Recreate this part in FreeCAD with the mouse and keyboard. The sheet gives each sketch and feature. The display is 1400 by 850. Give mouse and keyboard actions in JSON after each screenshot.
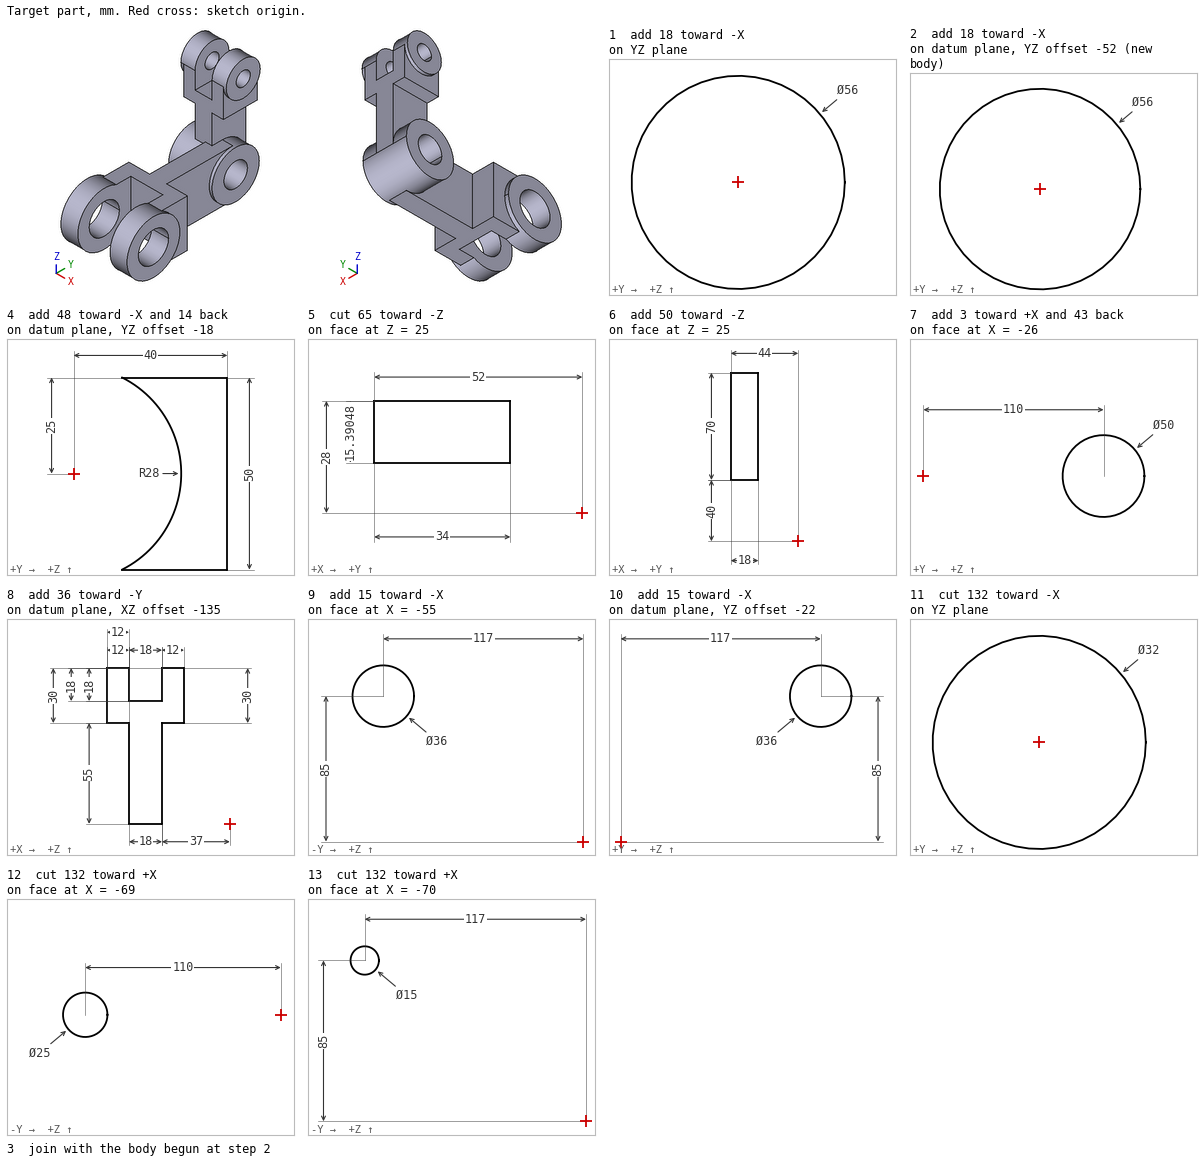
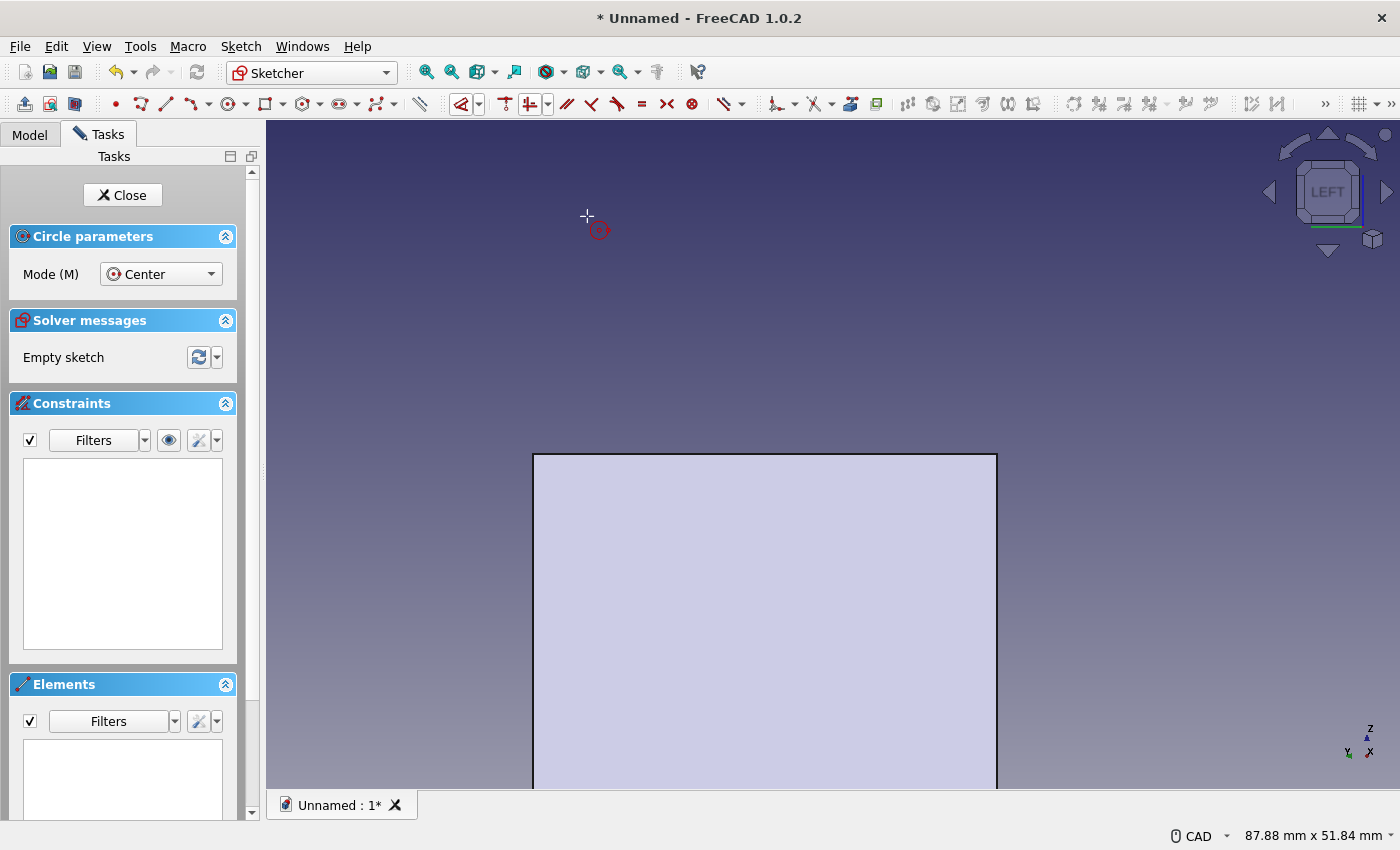
{"action": "left_click", "coordinate": [765, 454]}
{"action": "left_click", "coordinate": [929, 290]}
{"action": "key", "text": "Escape"}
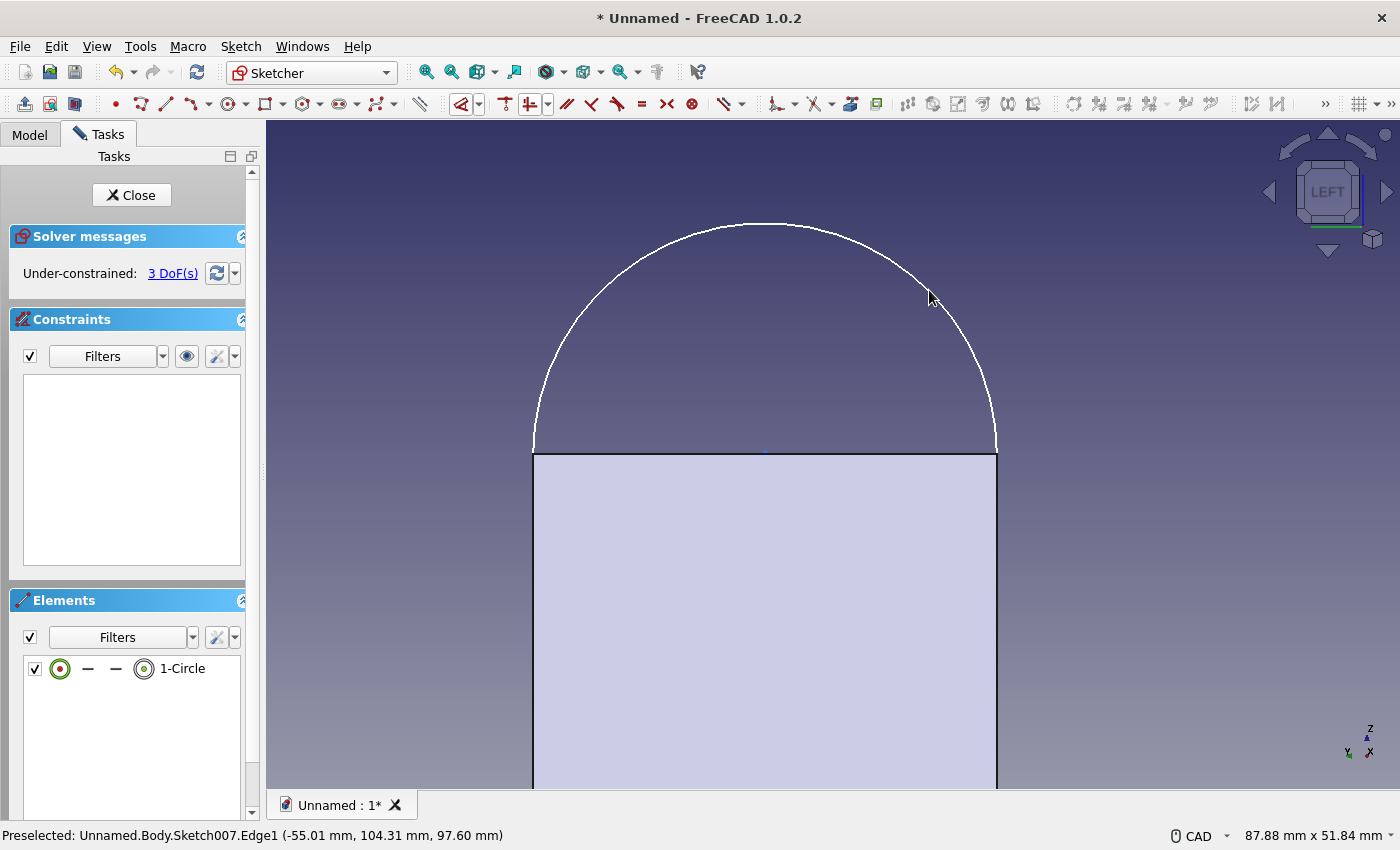
{"action": "left_click", "coordinate": [928, 290]}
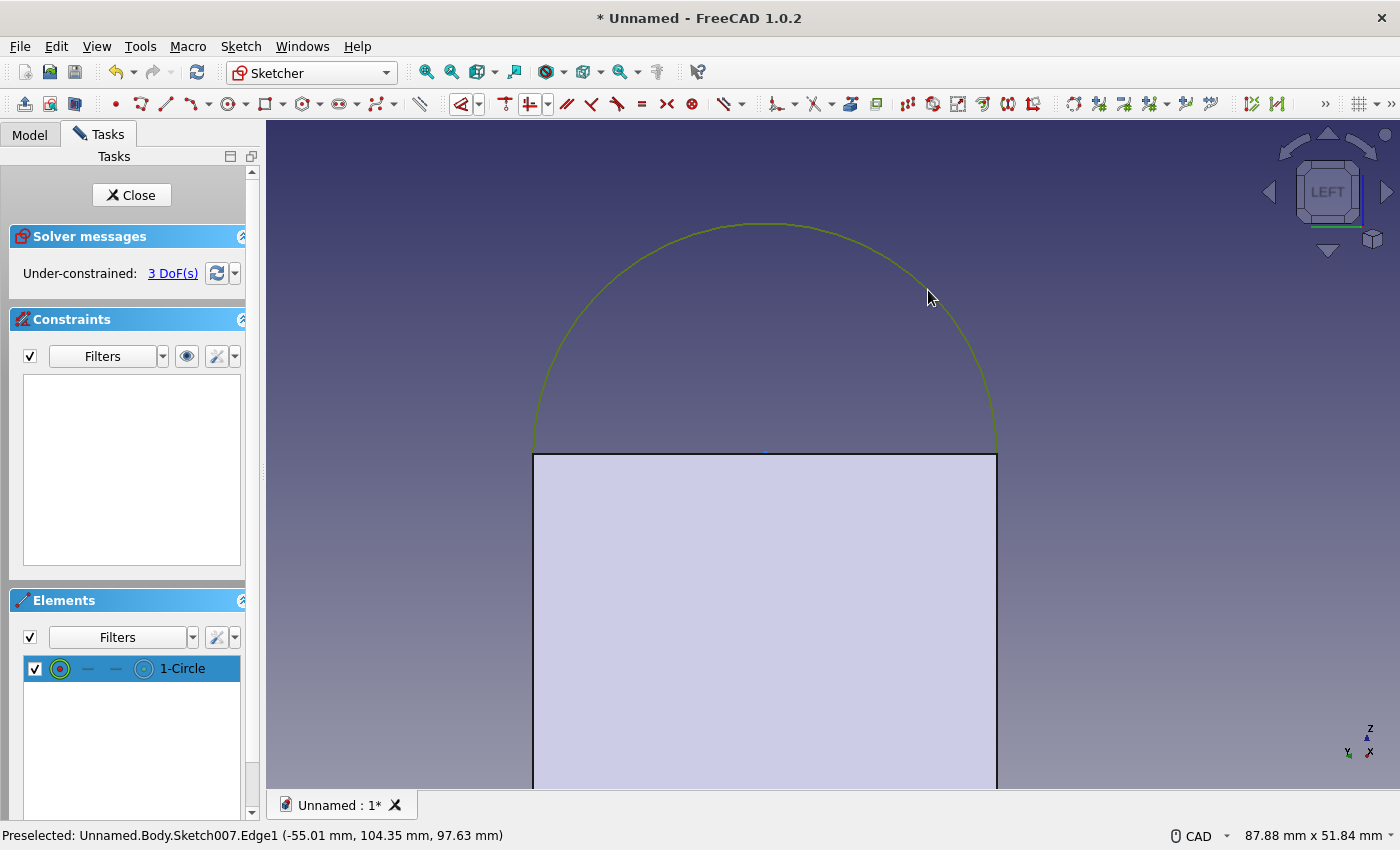
{"action": "key", "text": "k o"}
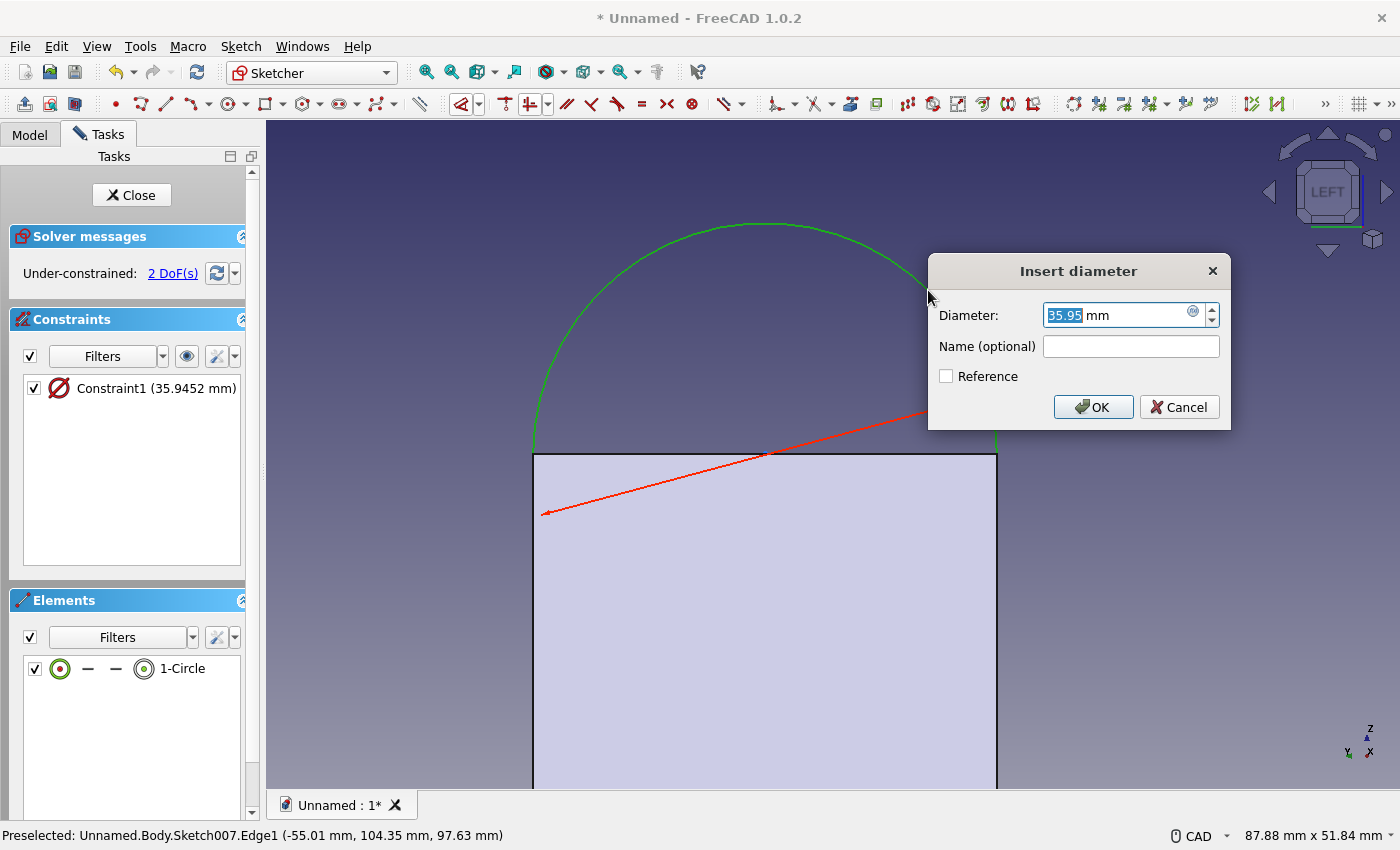
{"action": "type", "text": "36"}
{"action": "key", "text": "Return"}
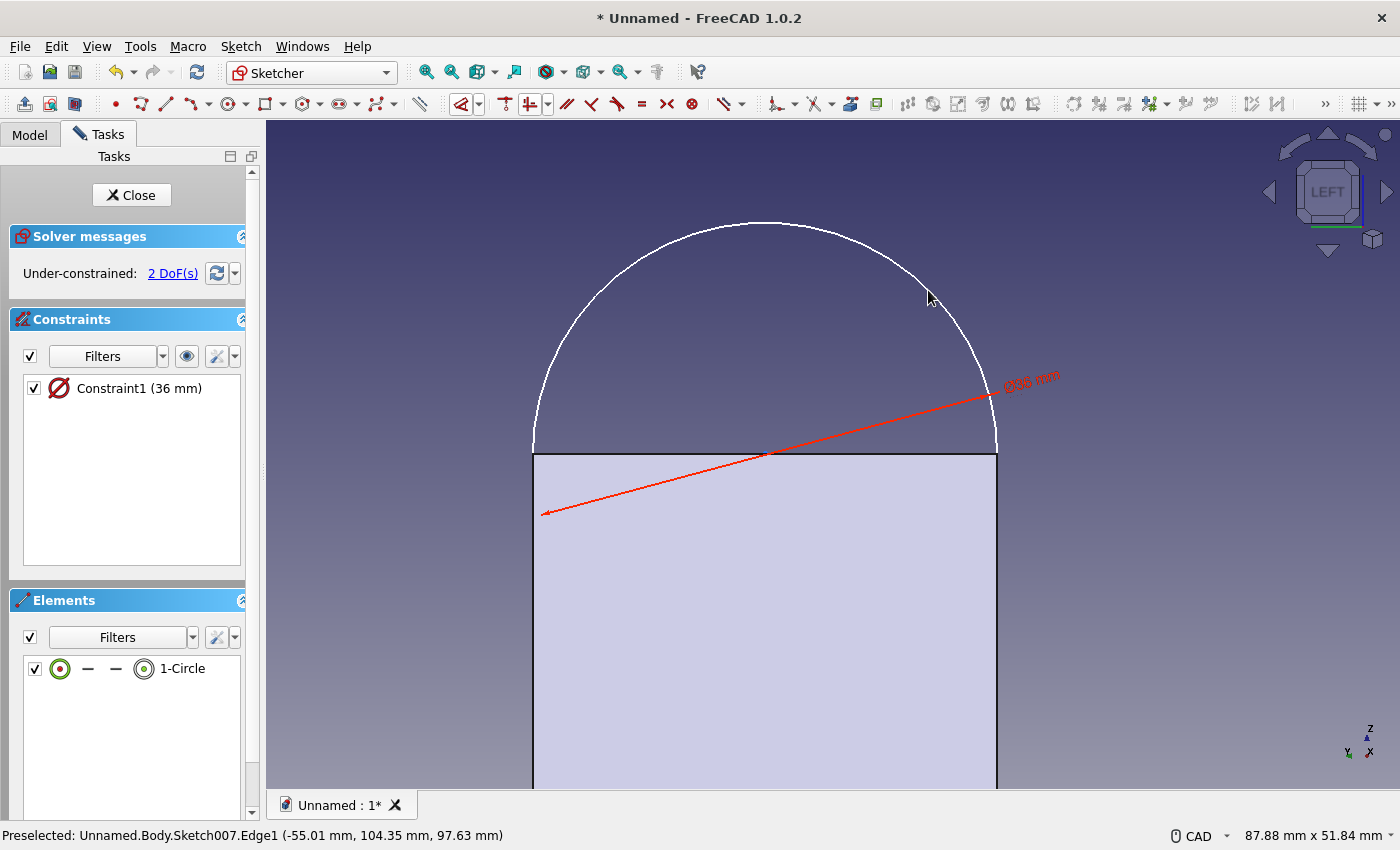
{"action": "left_click", "coordinate": [765, 455]}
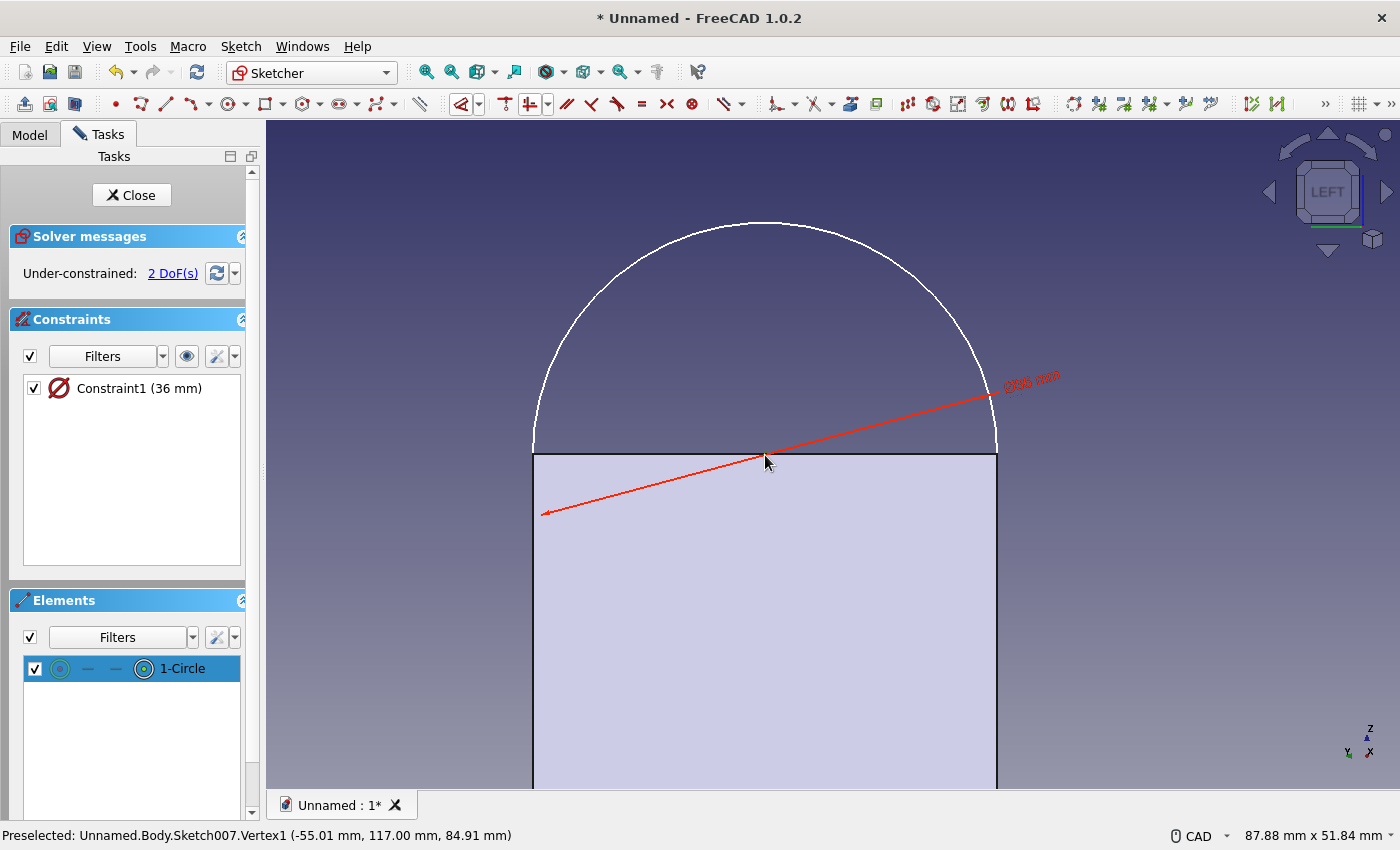
{"action": "key", "text": "i"}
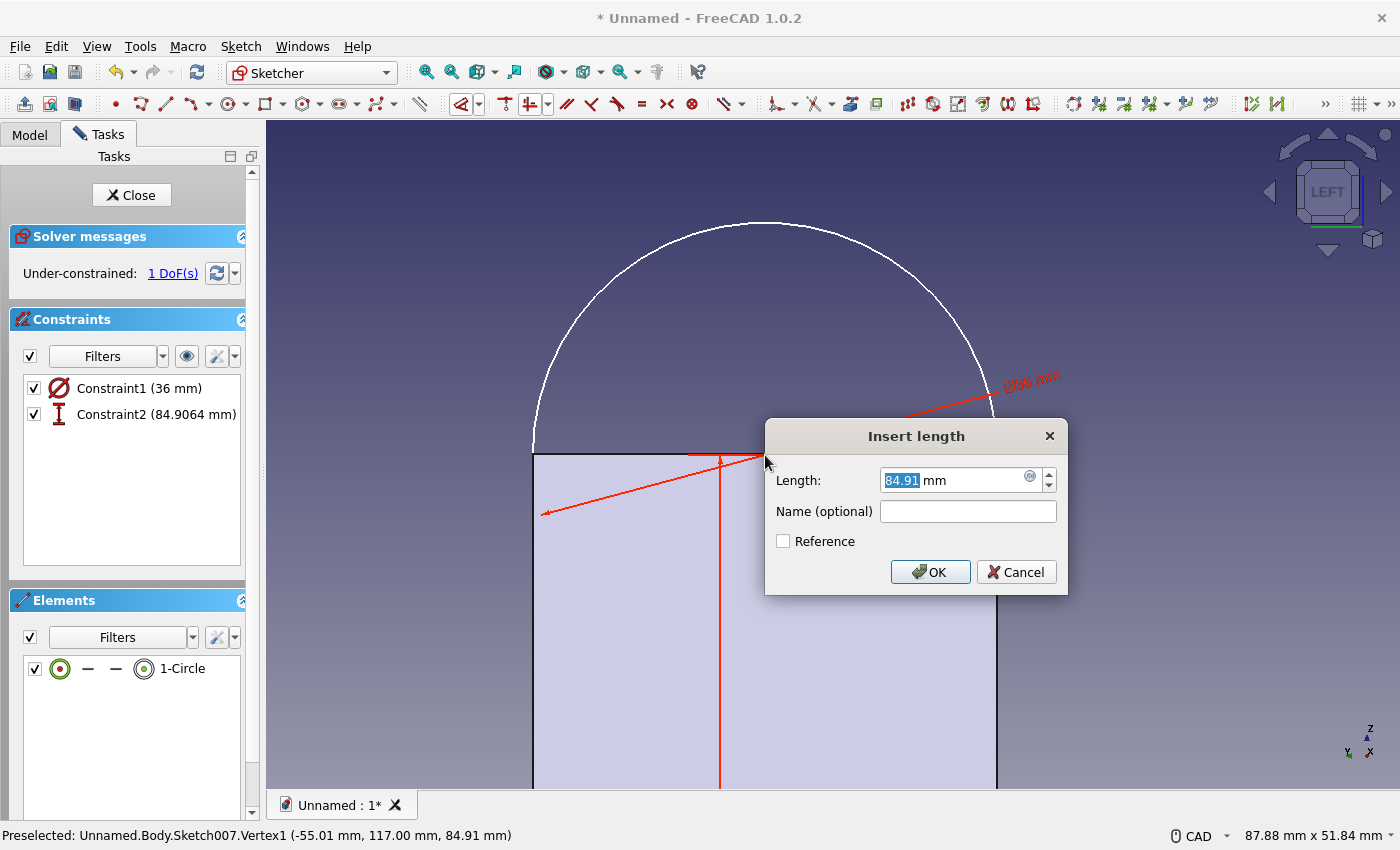
{"action": "type", "text": "85"}
{"action": "key", "text": "Return"}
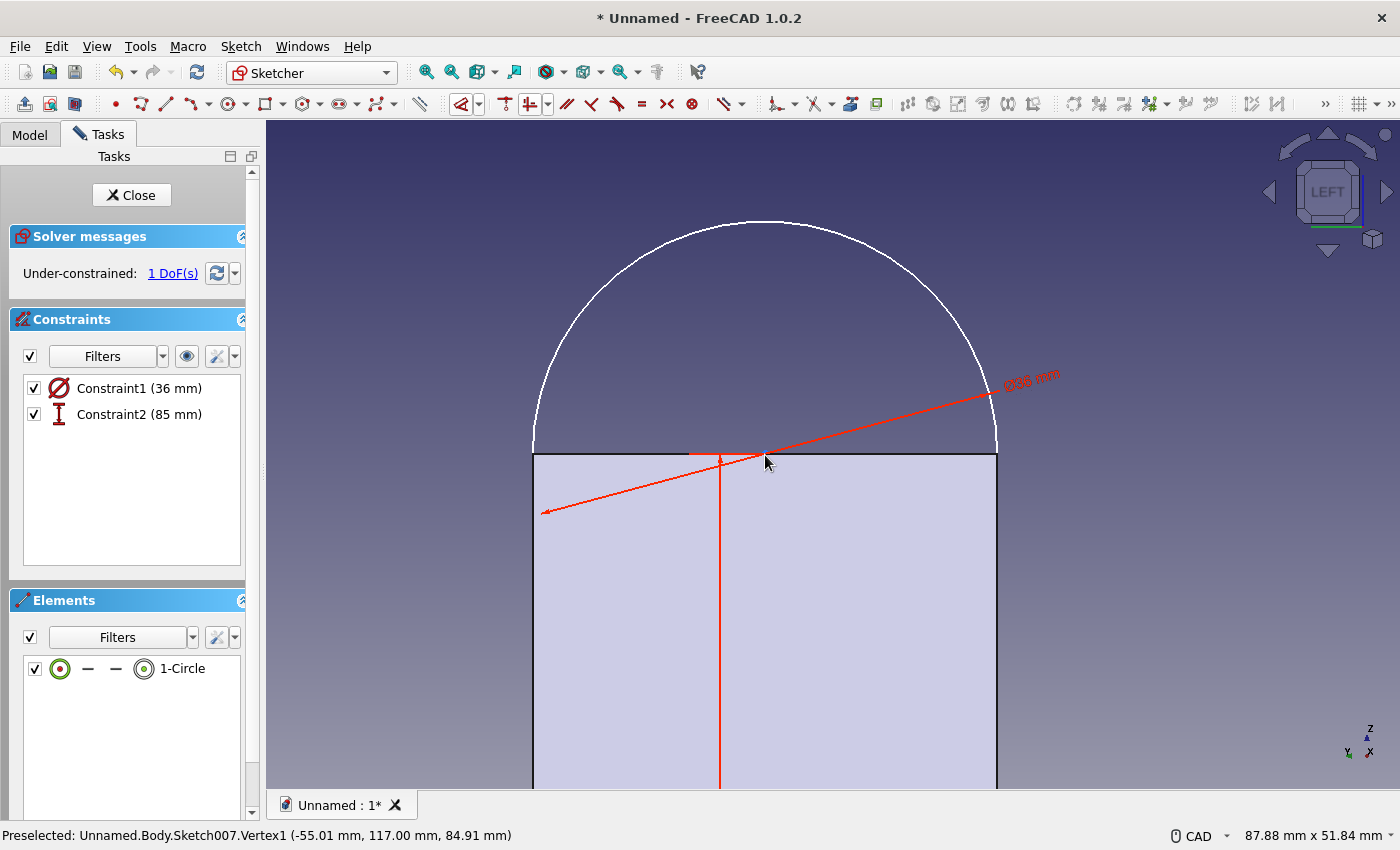
{"action": "left_click", "coordinate": [765, 454]}